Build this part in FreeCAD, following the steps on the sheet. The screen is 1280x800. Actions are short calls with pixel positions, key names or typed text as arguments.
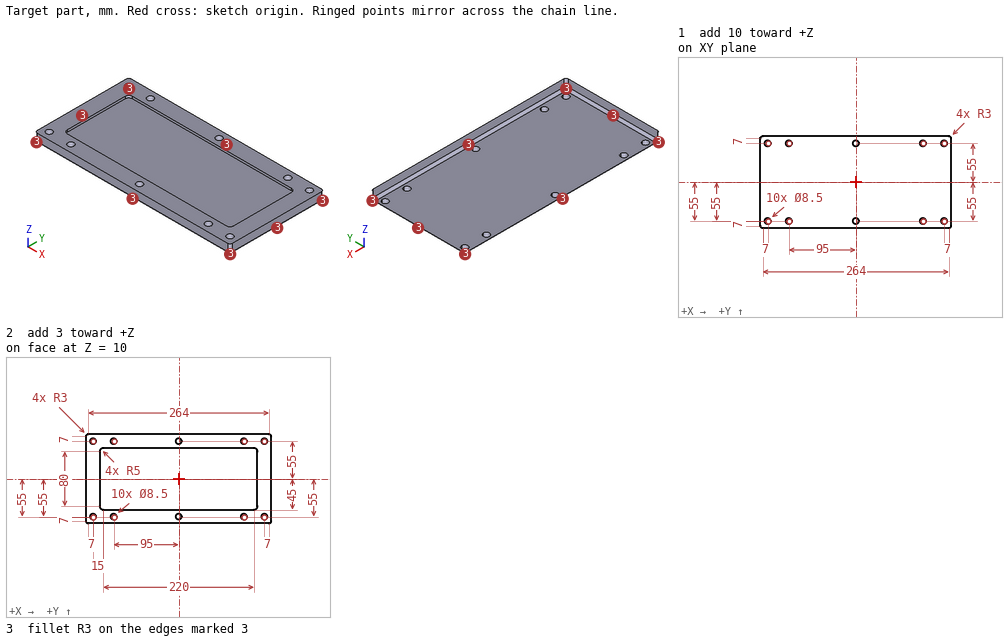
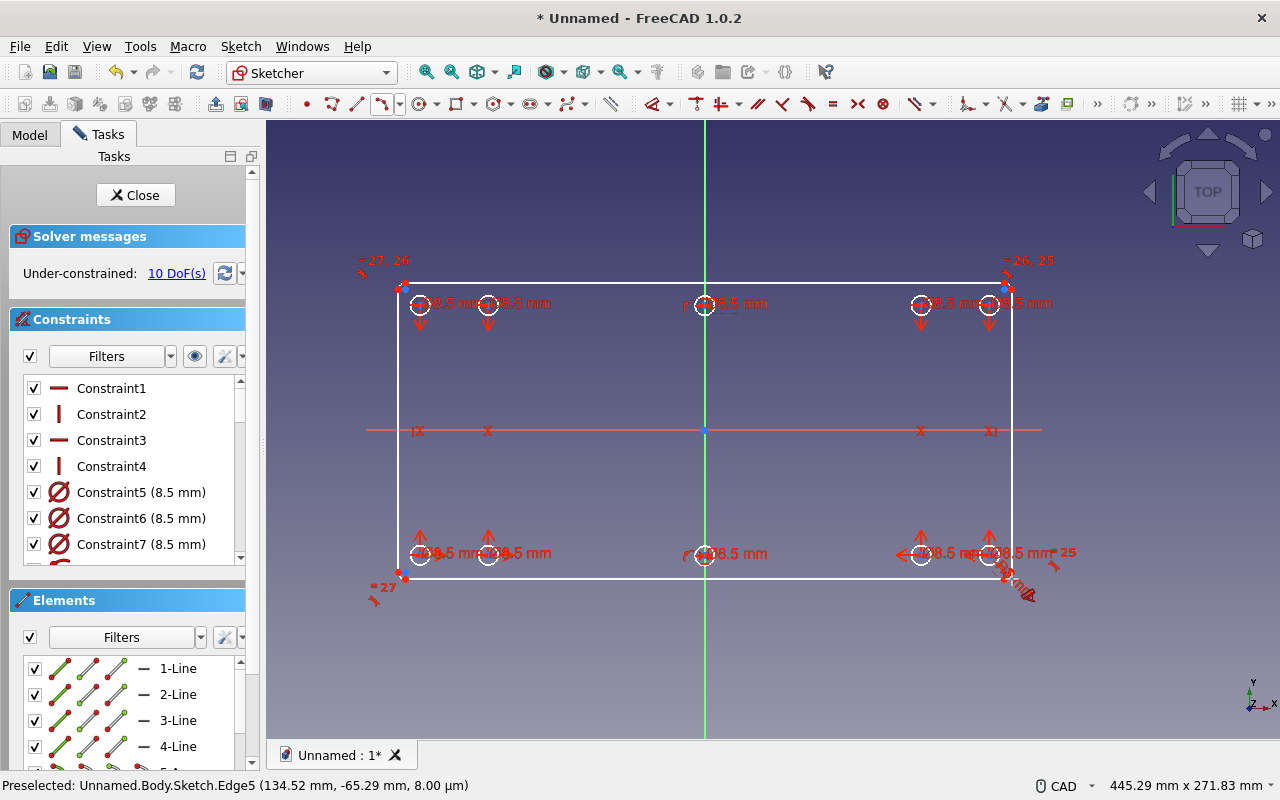
click(420, 555)
click(739, 493)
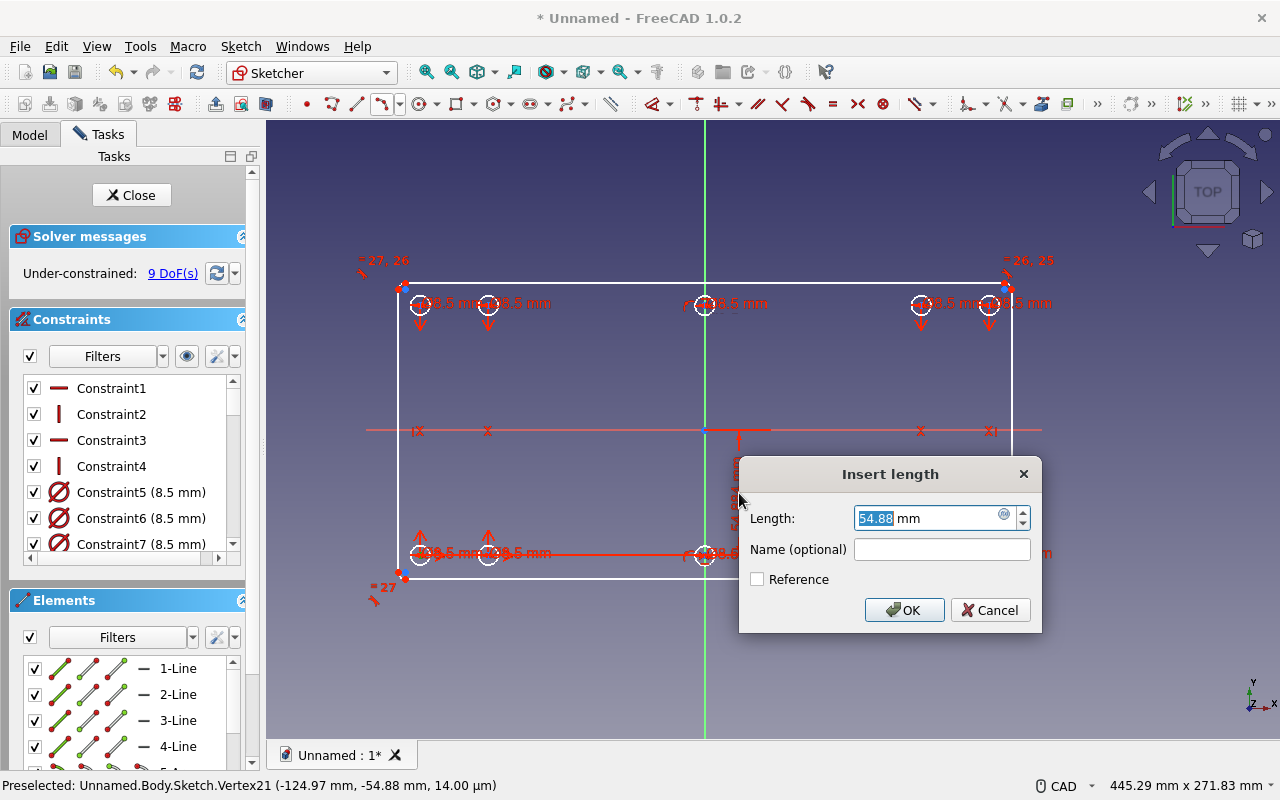
text(55)
key(Return)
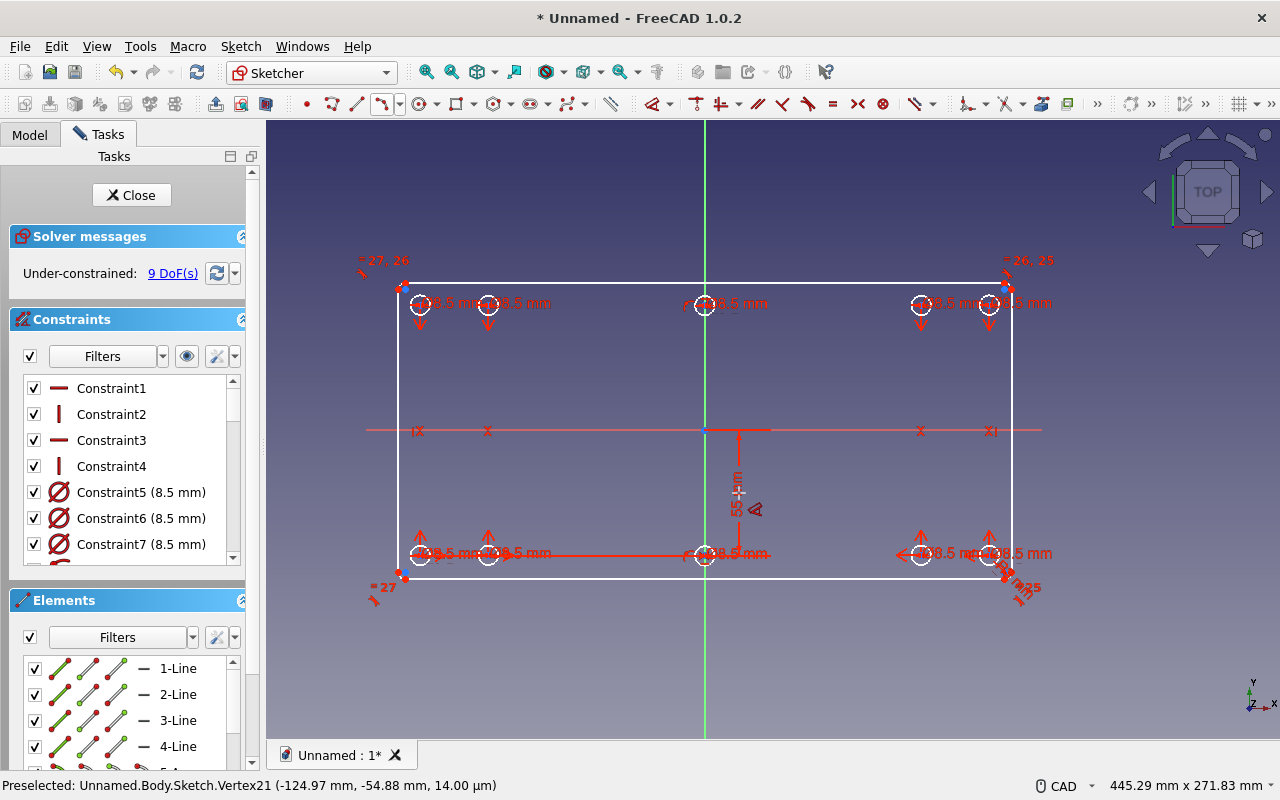
click(488, 555)
click(597, 396)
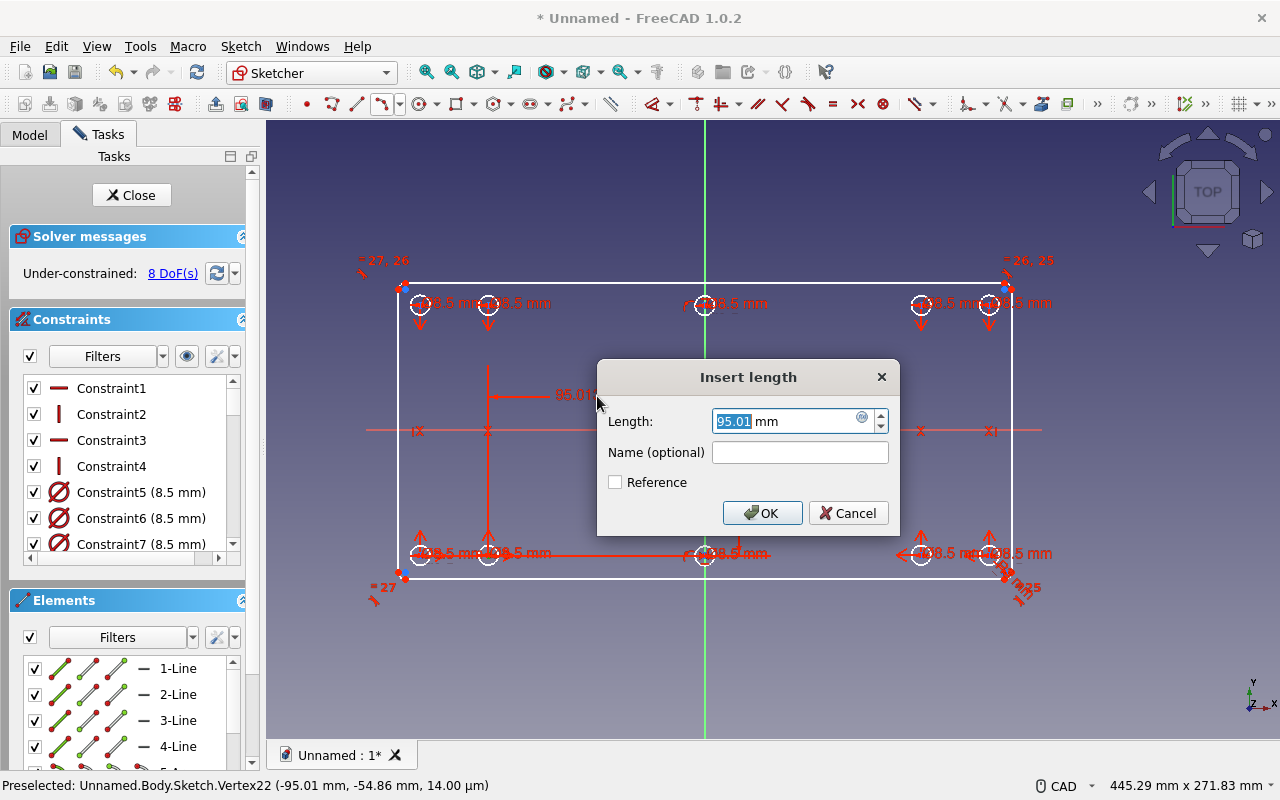
text(95)
key(Return)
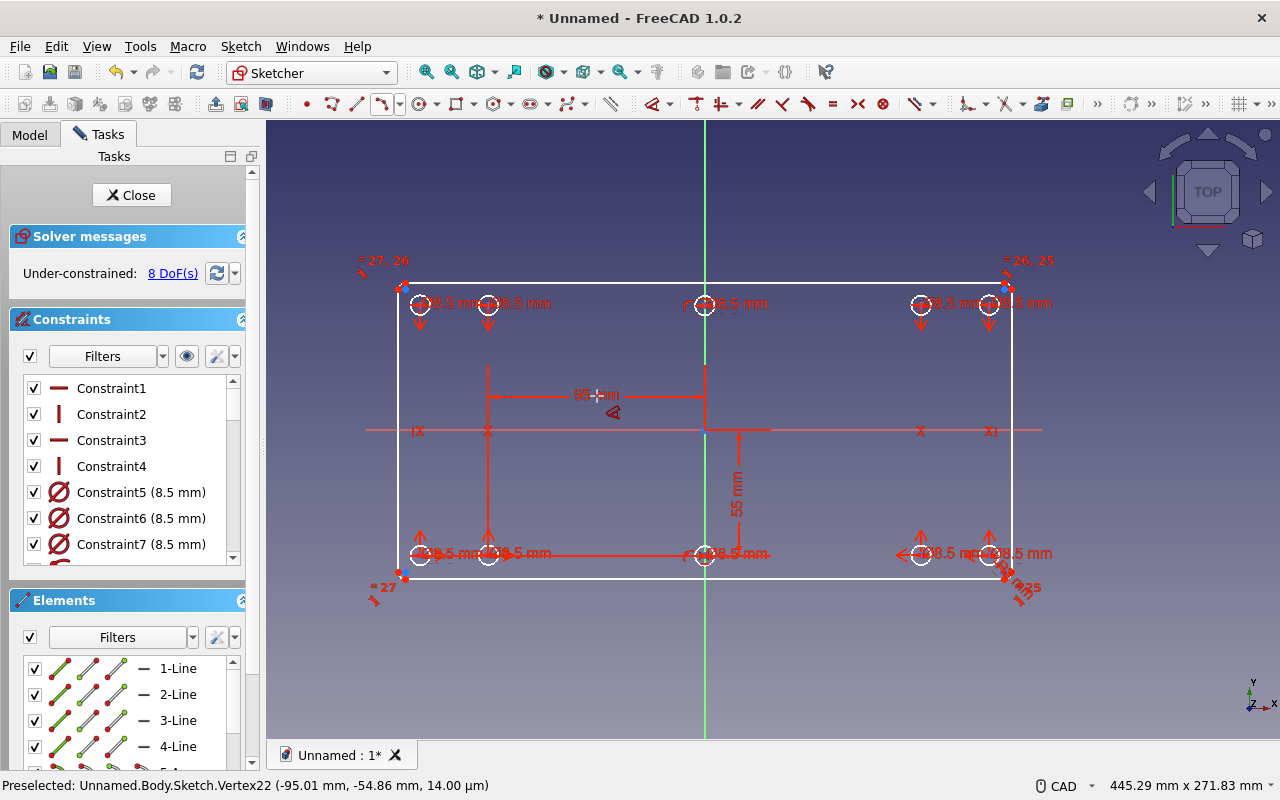
click(488, 555)
click(454, 493)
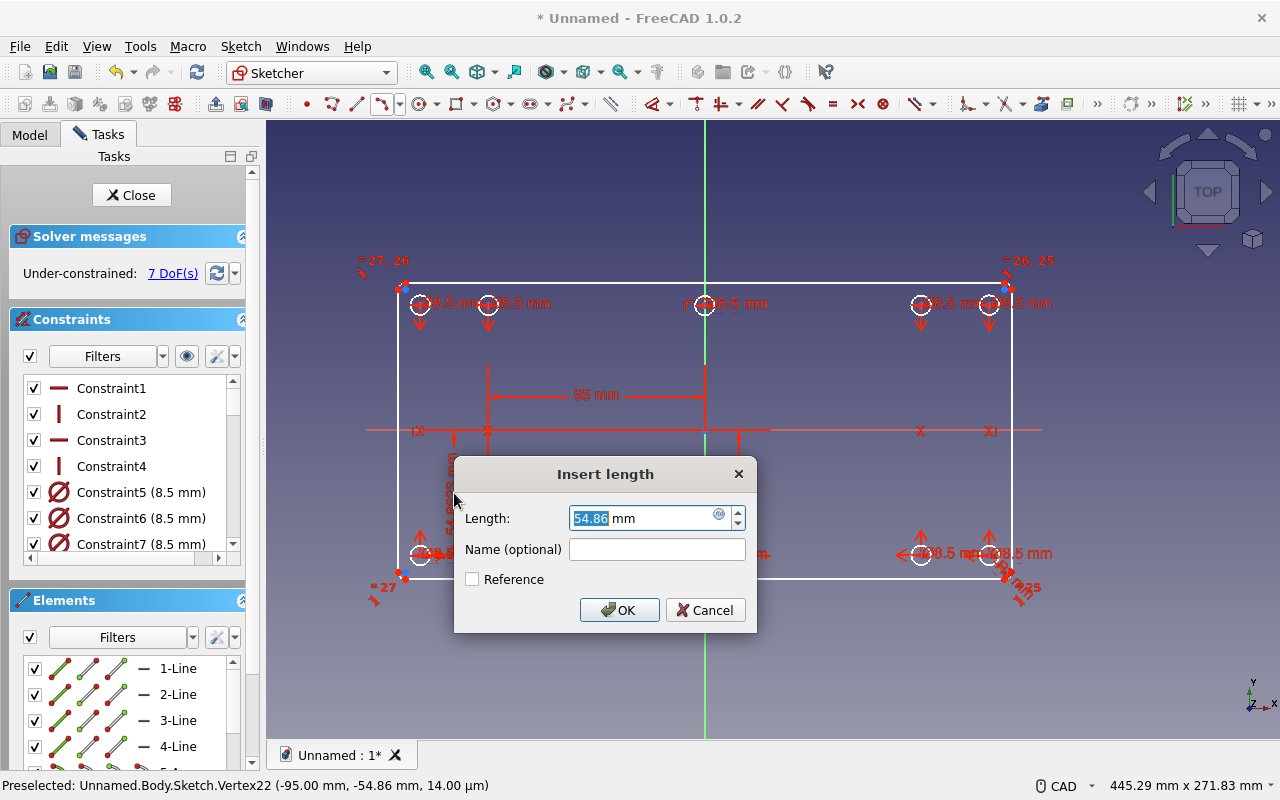
text(55)
key(Return)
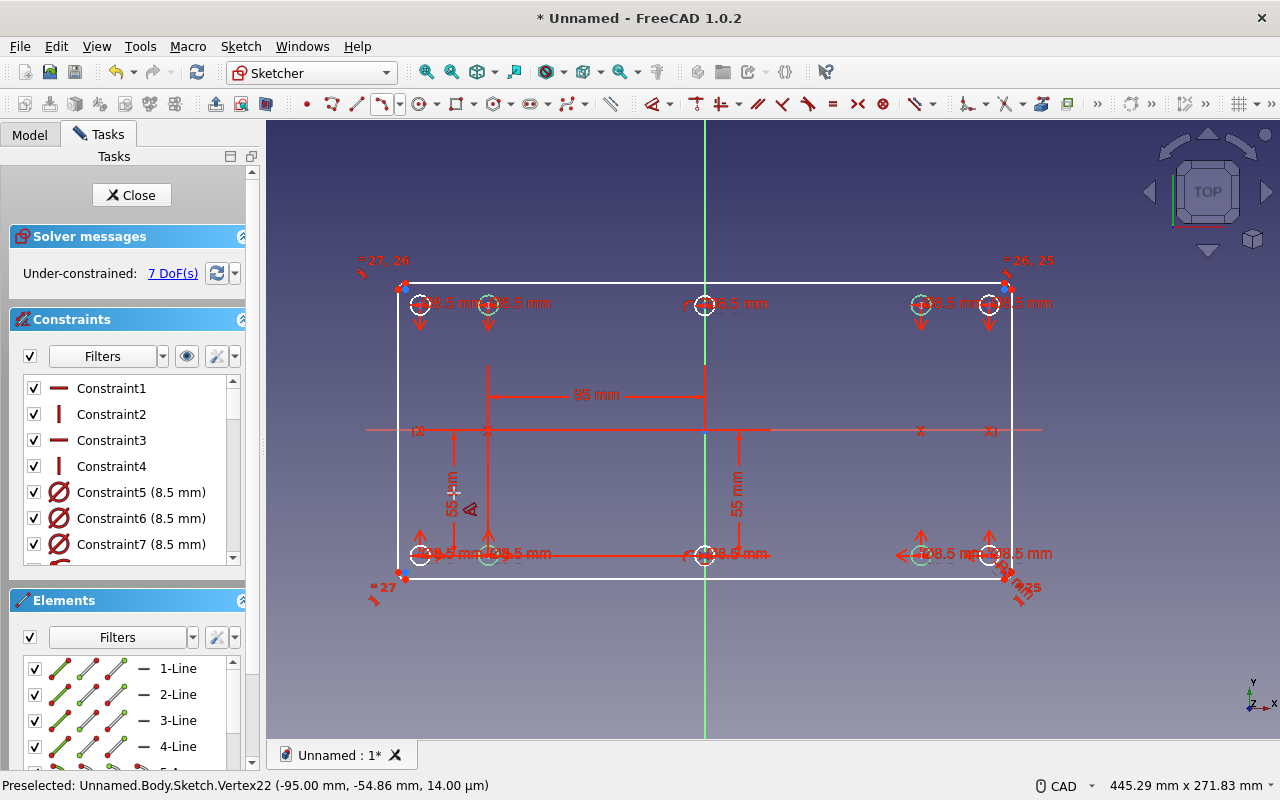
click(705, 556)
click(739, 464)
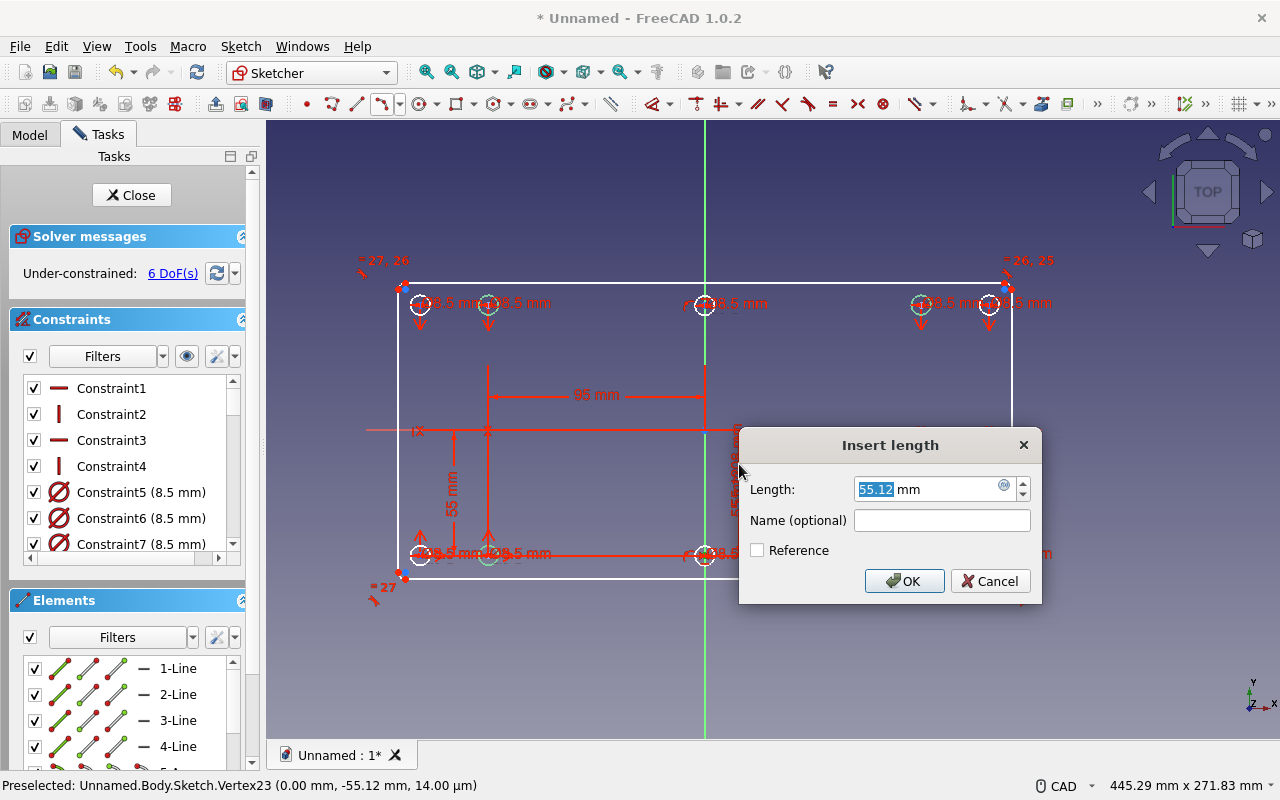
text(55)
key(Return)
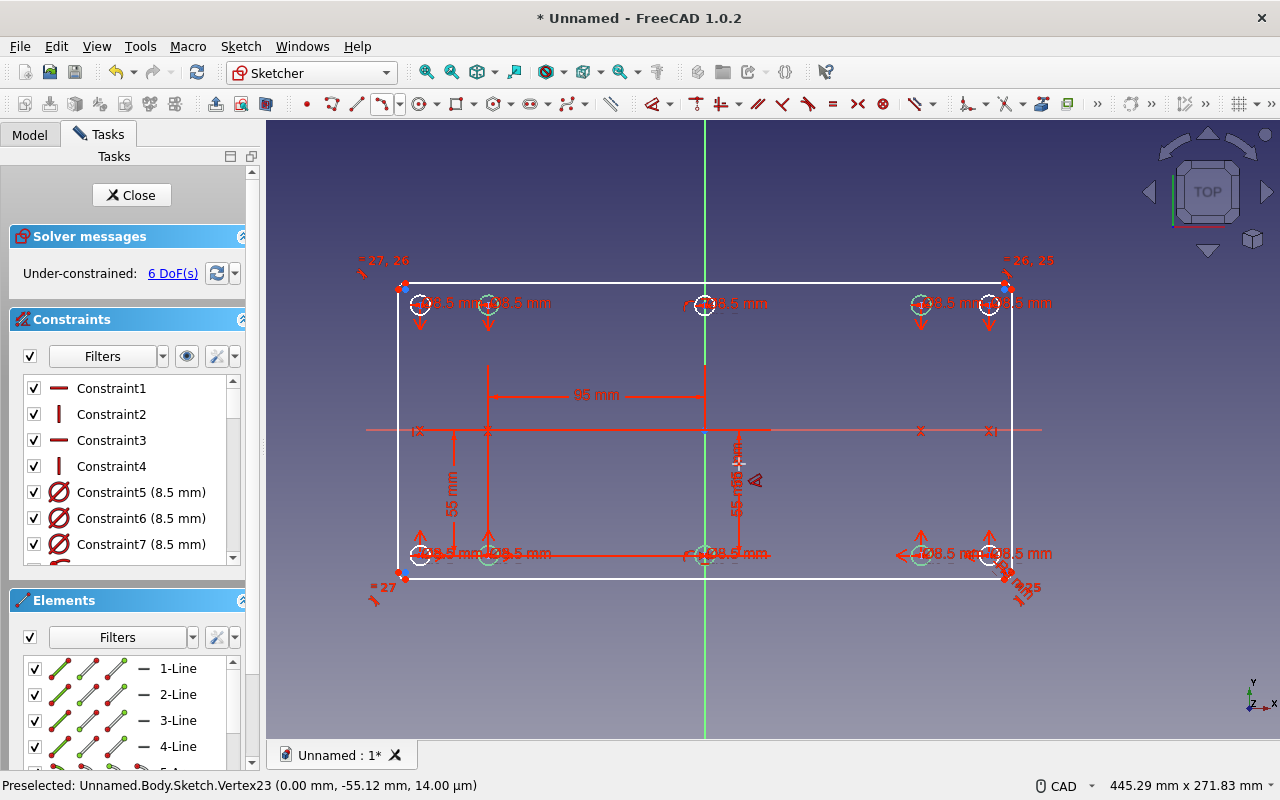
click(705, 306)
click(739, 368)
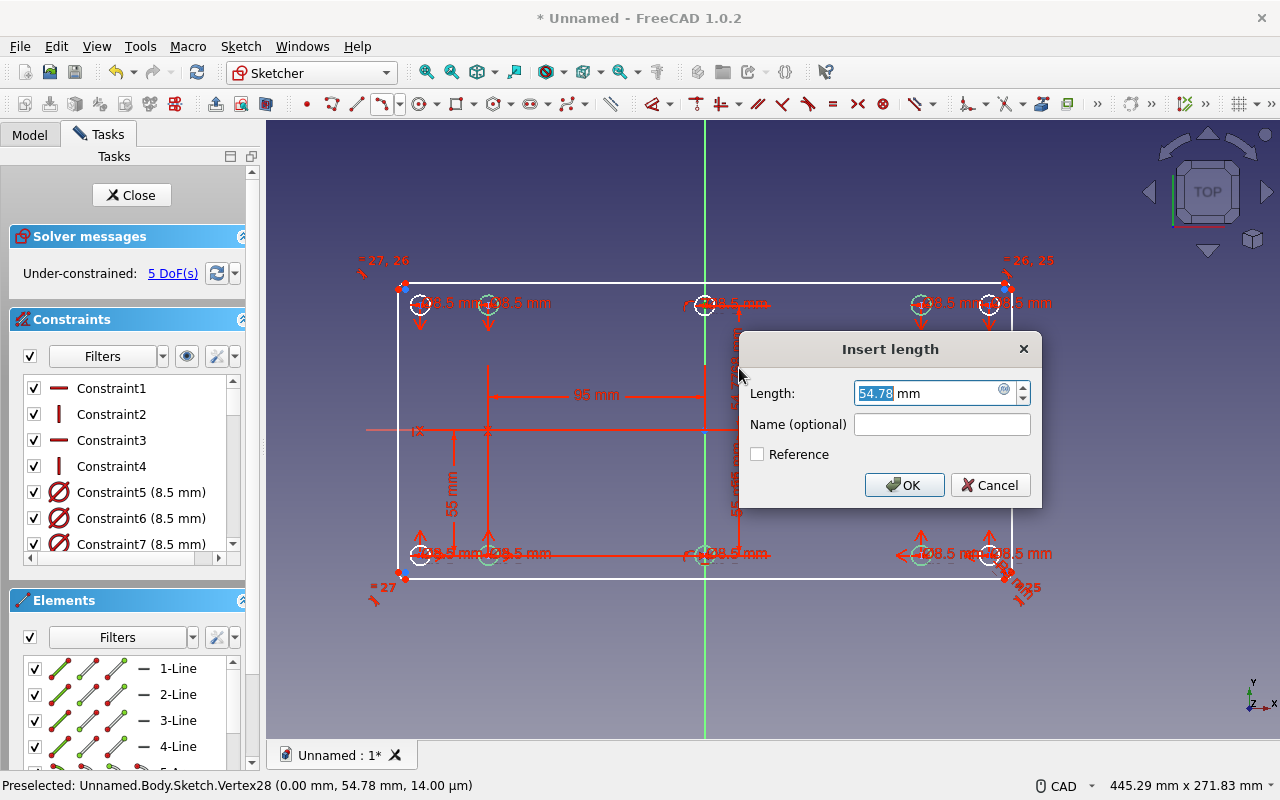
text(55)
key(Return)